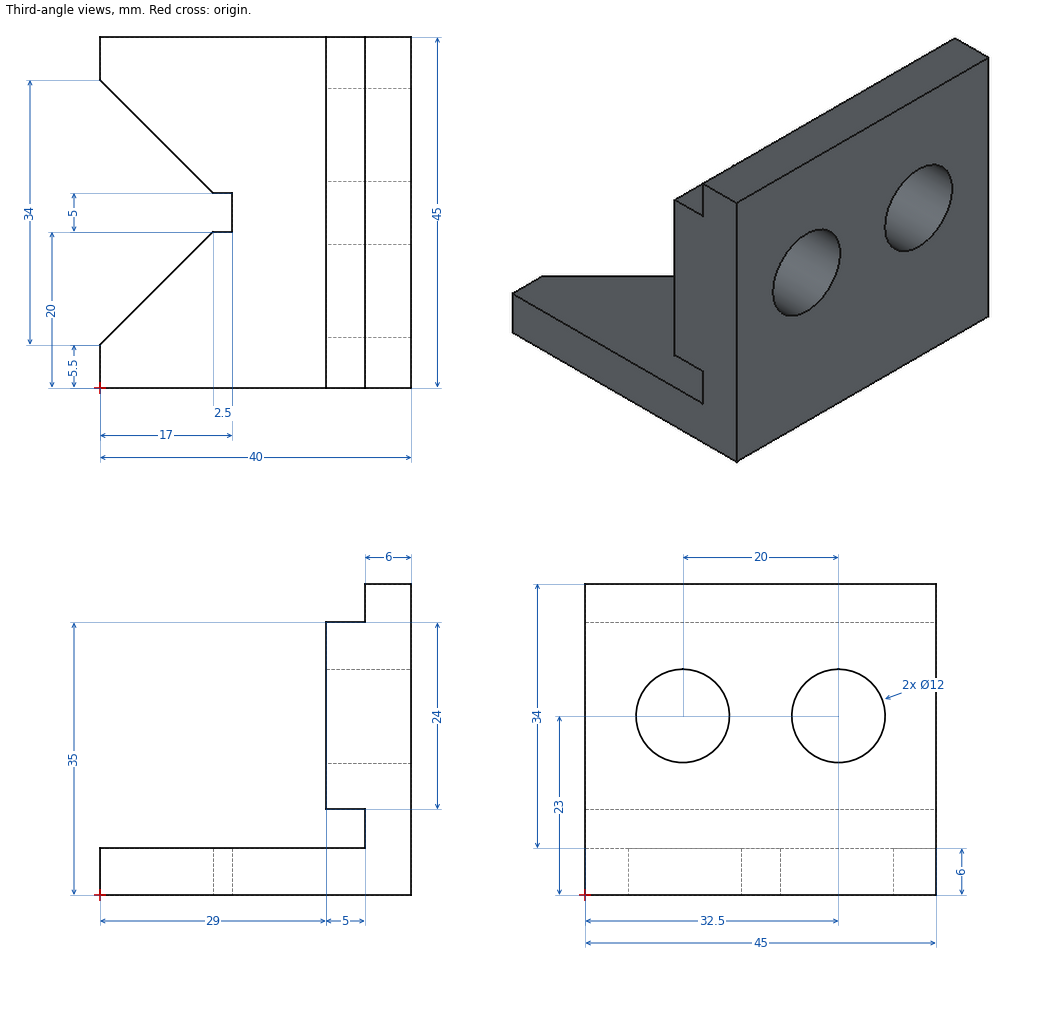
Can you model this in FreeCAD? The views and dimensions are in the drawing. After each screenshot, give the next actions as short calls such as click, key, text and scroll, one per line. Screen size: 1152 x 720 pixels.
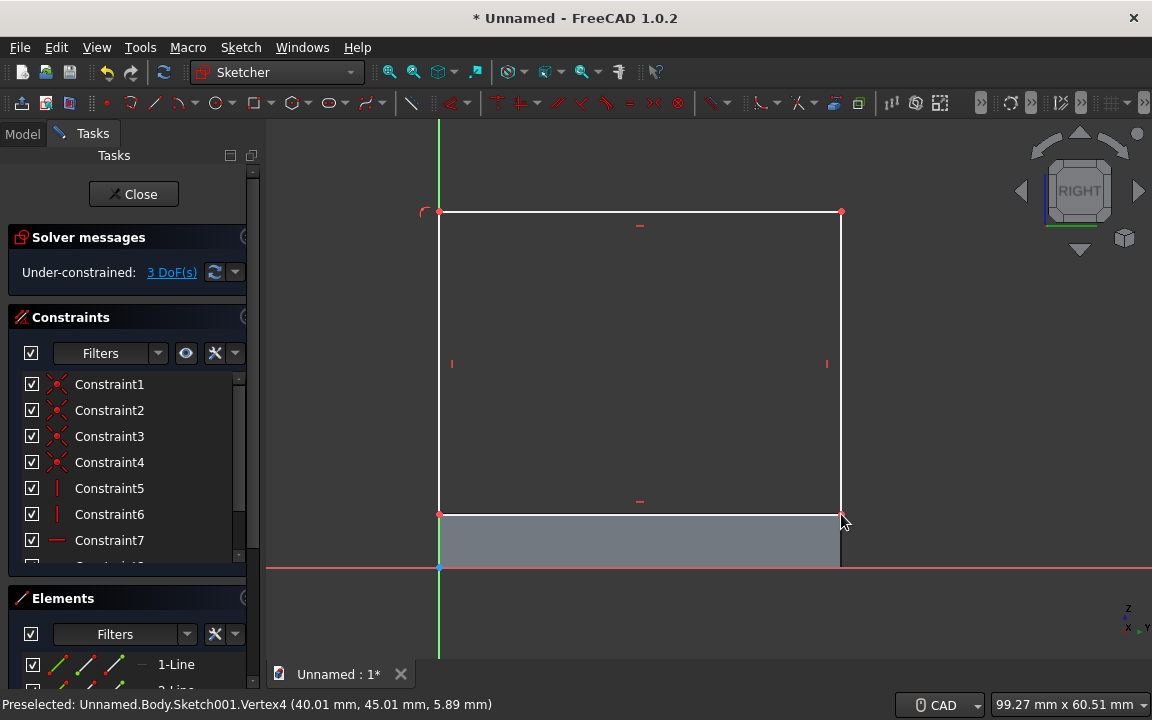
click(450, 104)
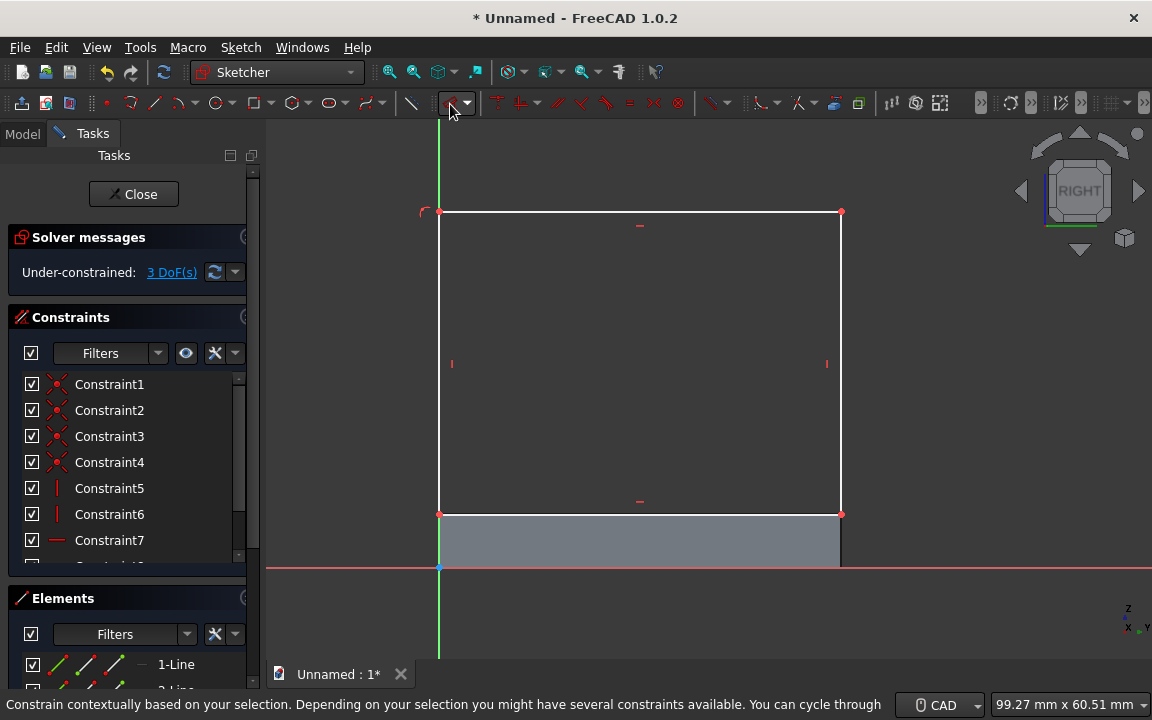
click(439, 303)
click(405, 363)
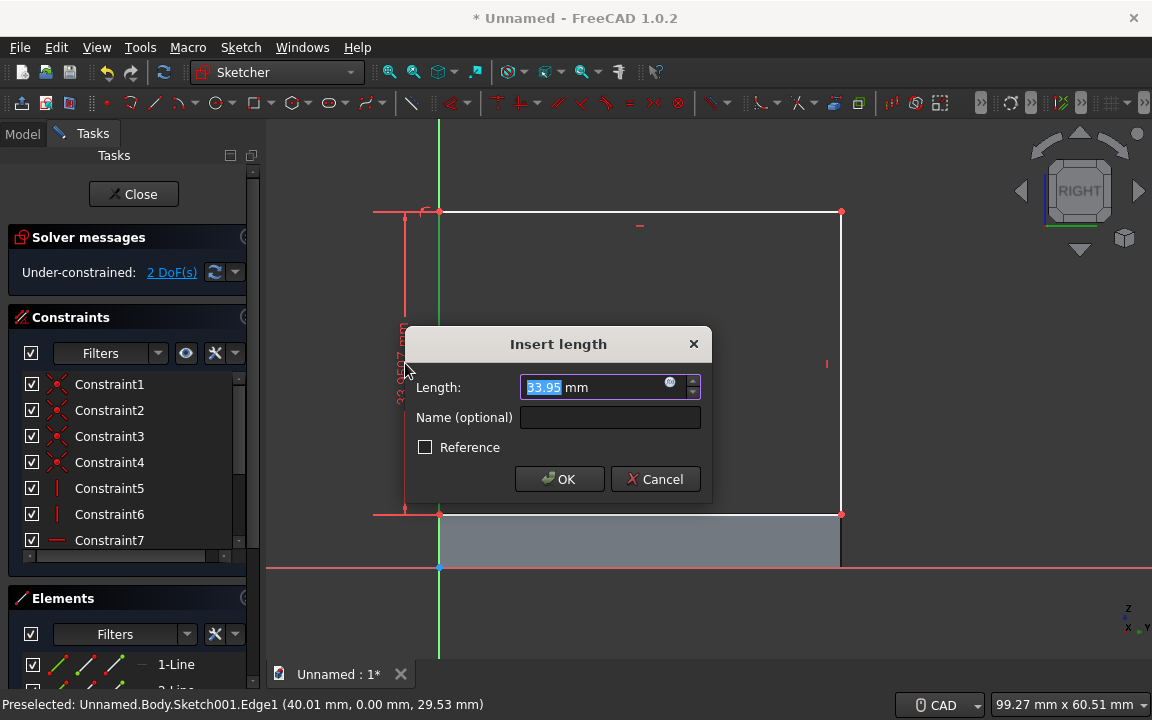
text(34)
key(Return)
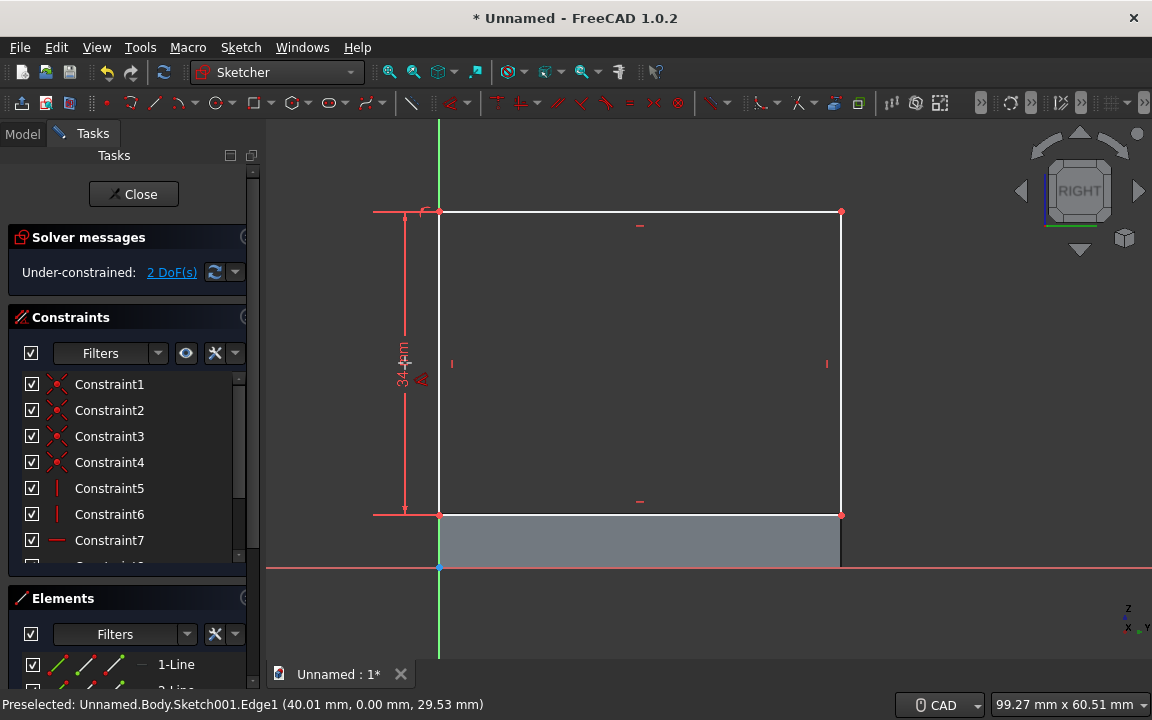
click(560, 515)
click(640, 549)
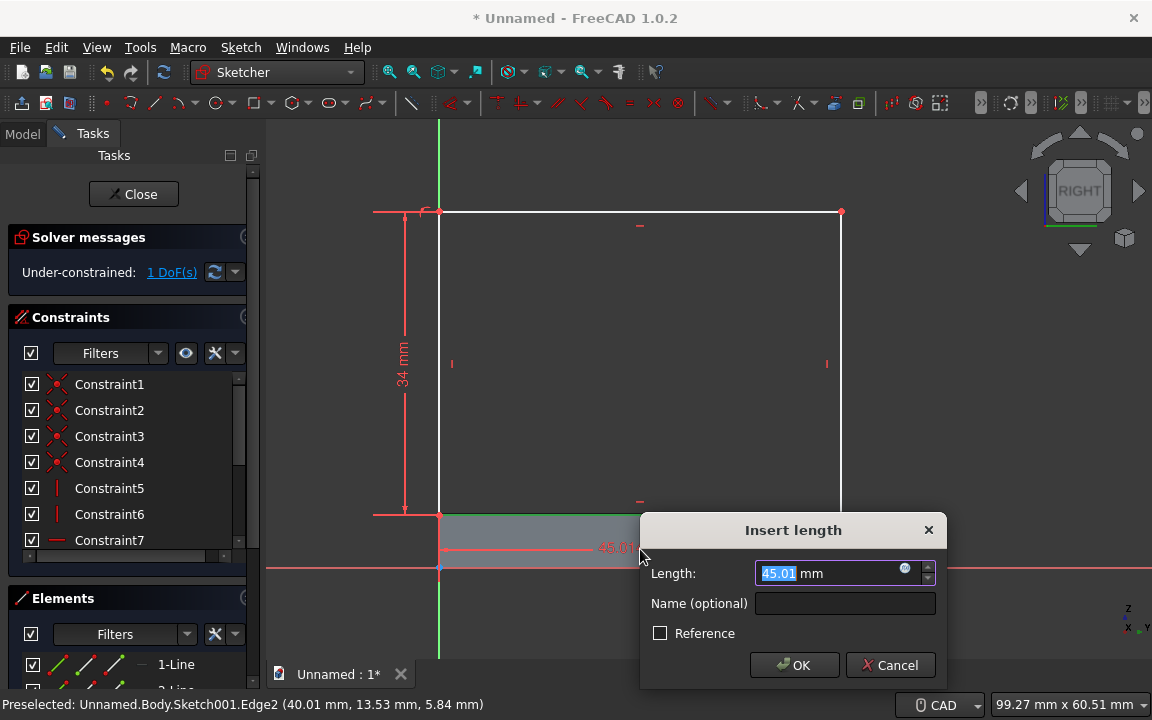
text(45)
key(Return)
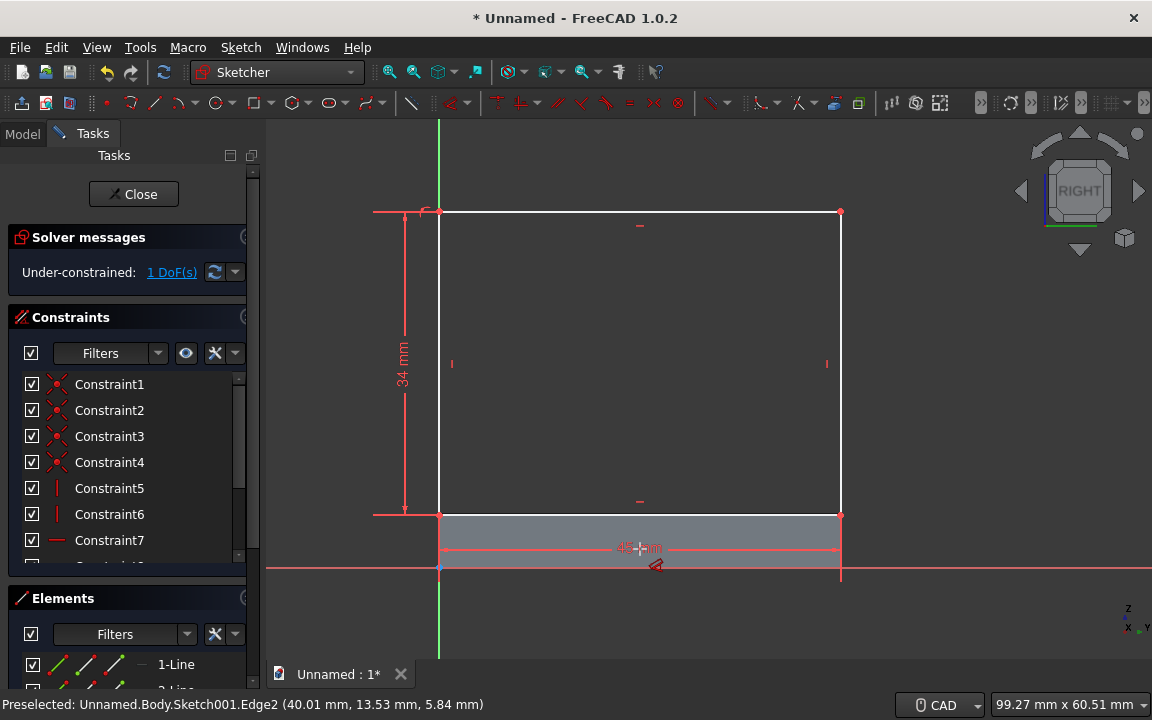
click(439, 515)
click(405, 541)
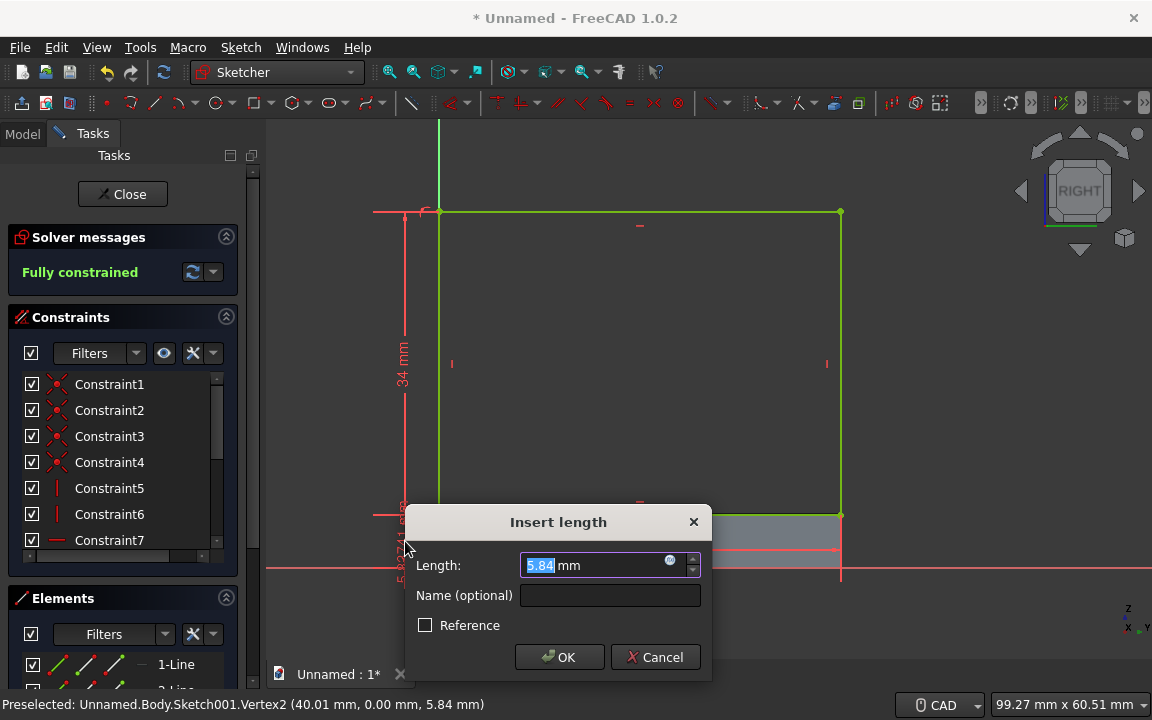
text(6)
key(Return)
key(Escape)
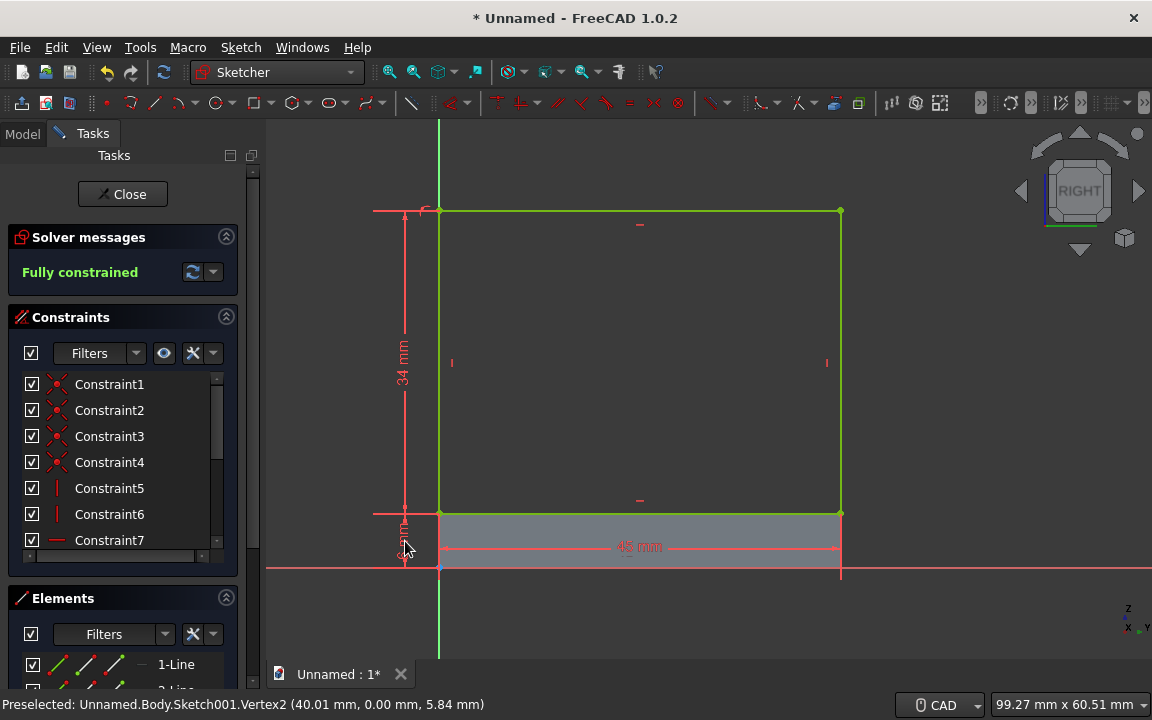
click(123, 194)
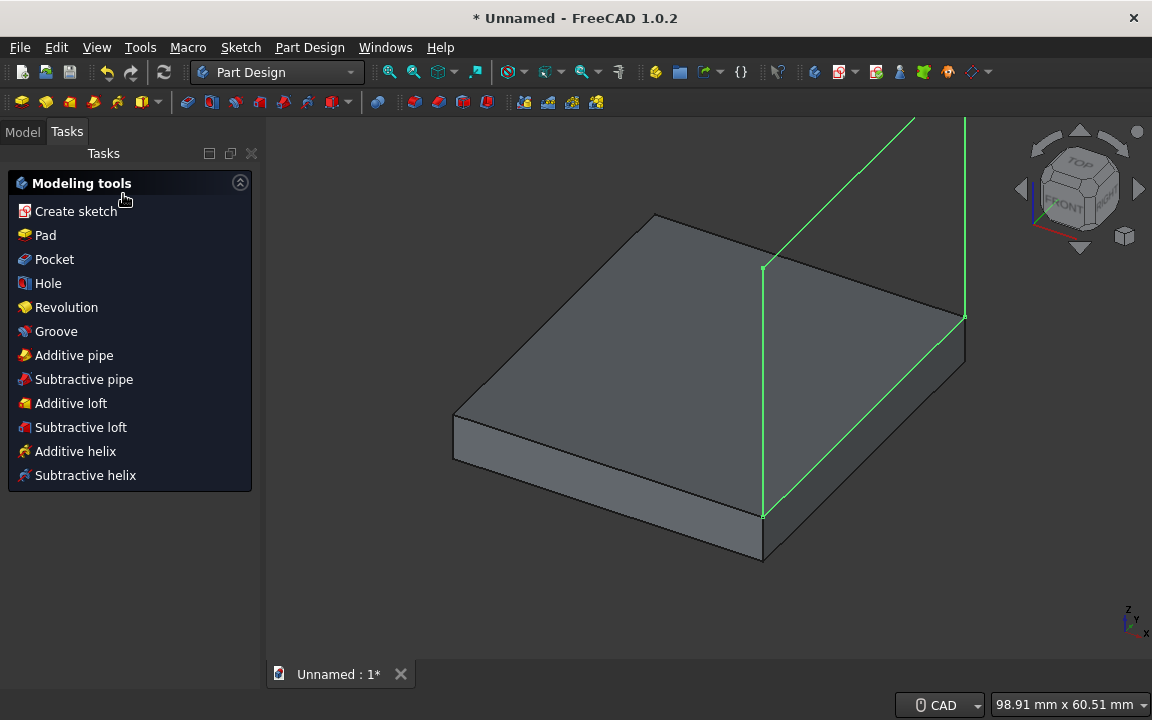
click(22, 102)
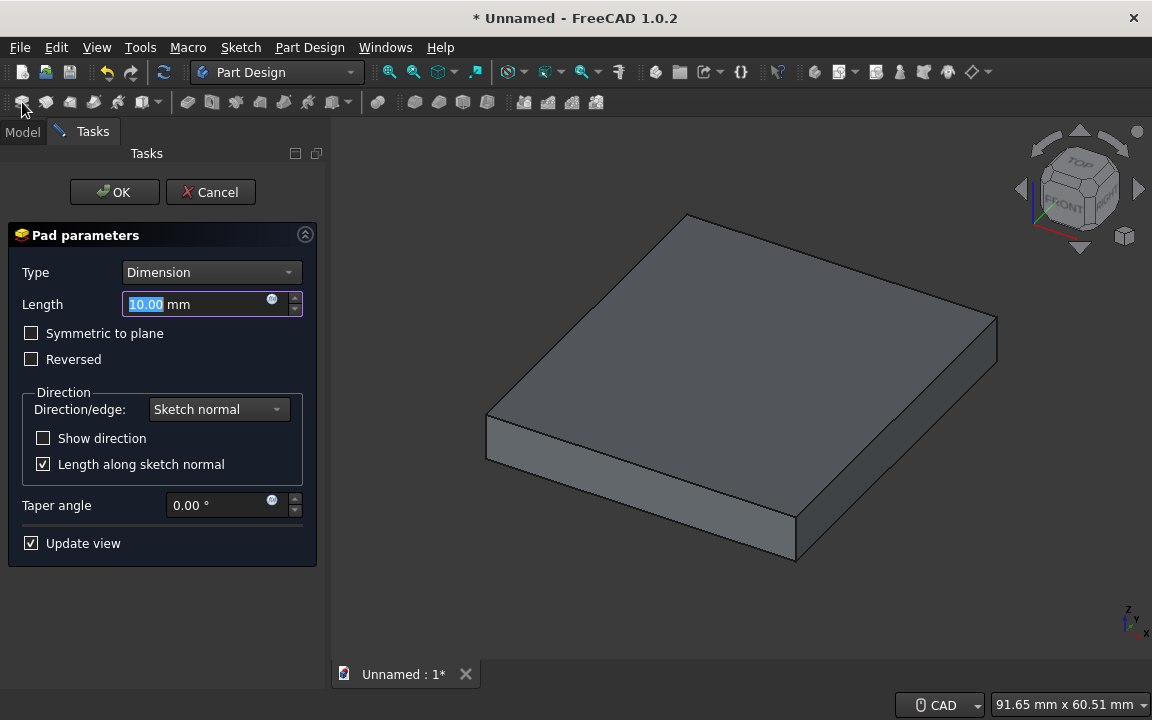
text(6)
key(Tab)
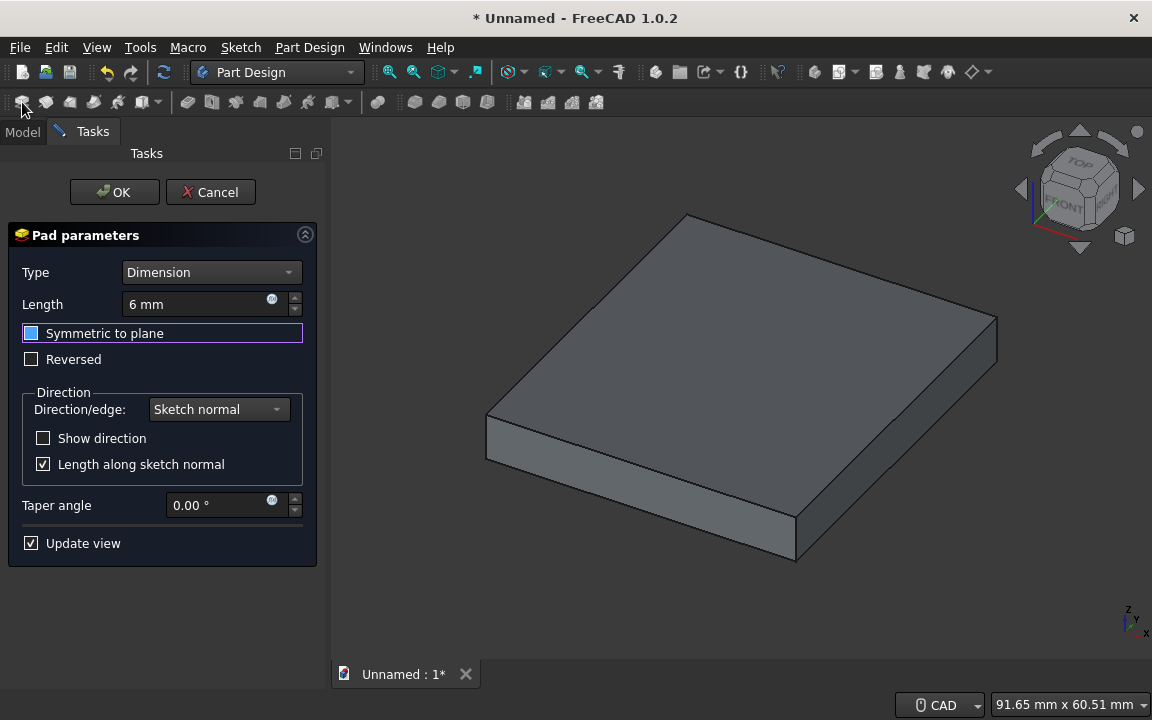
click(30, 359)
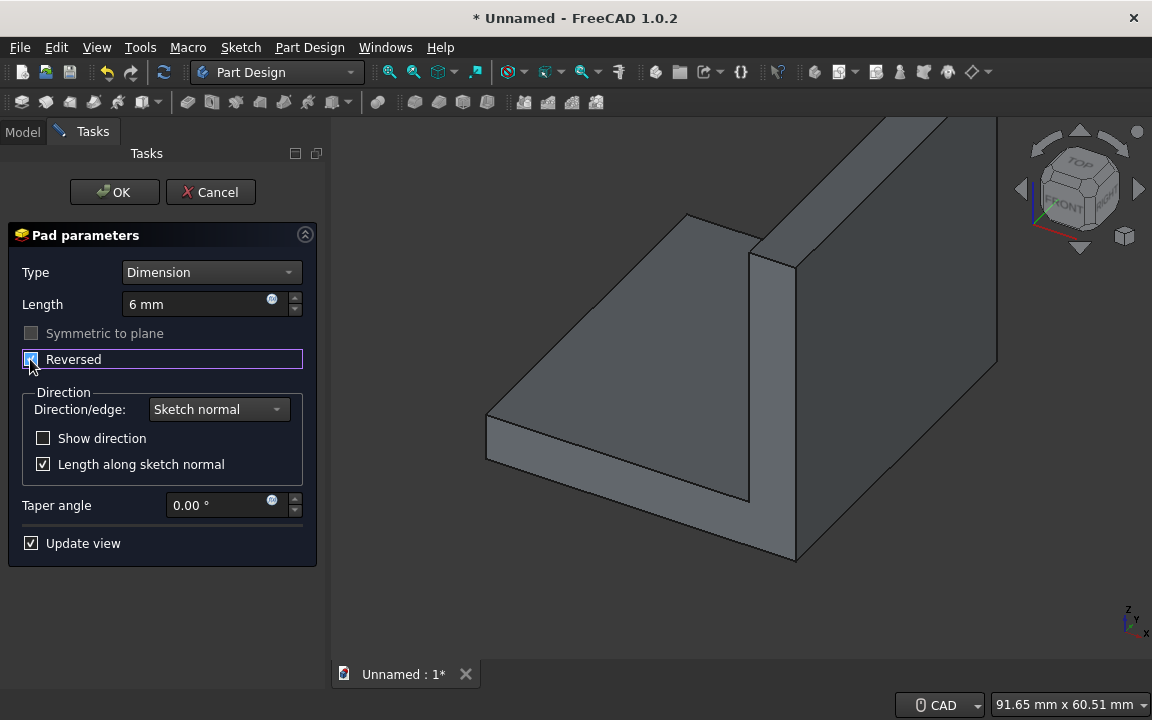
click(115, 192)